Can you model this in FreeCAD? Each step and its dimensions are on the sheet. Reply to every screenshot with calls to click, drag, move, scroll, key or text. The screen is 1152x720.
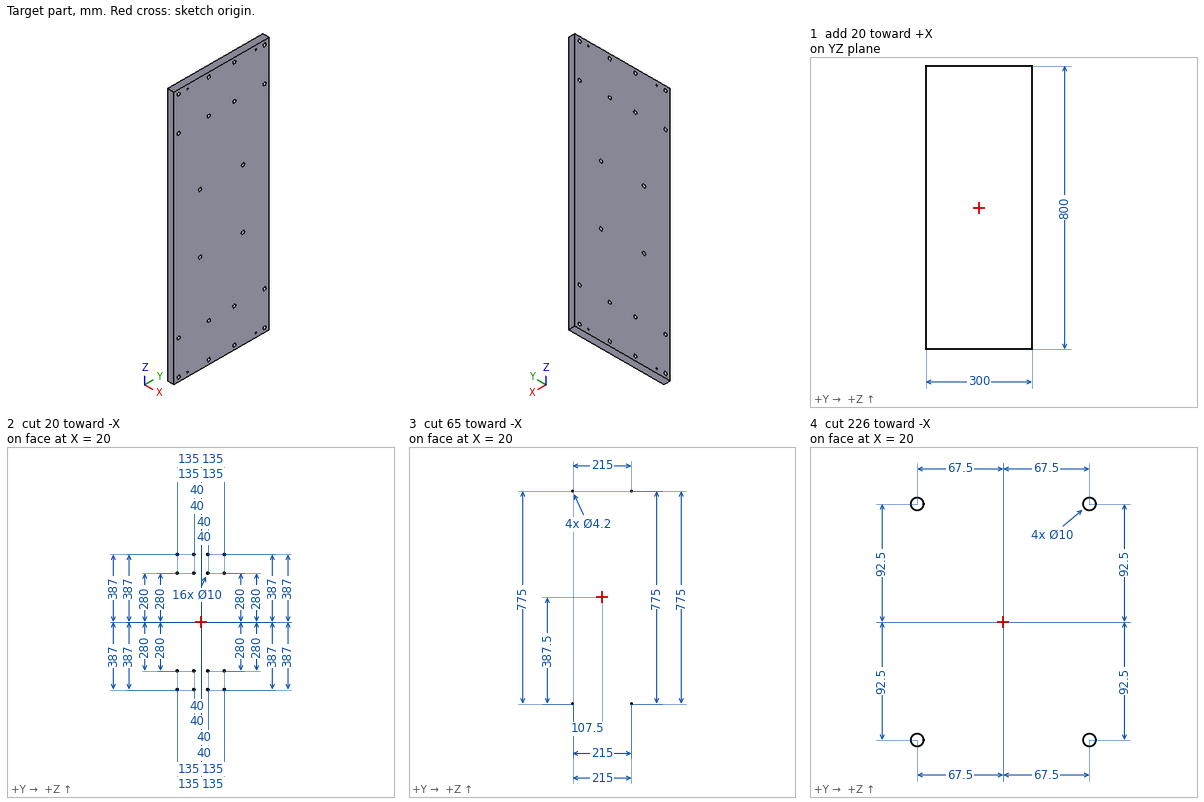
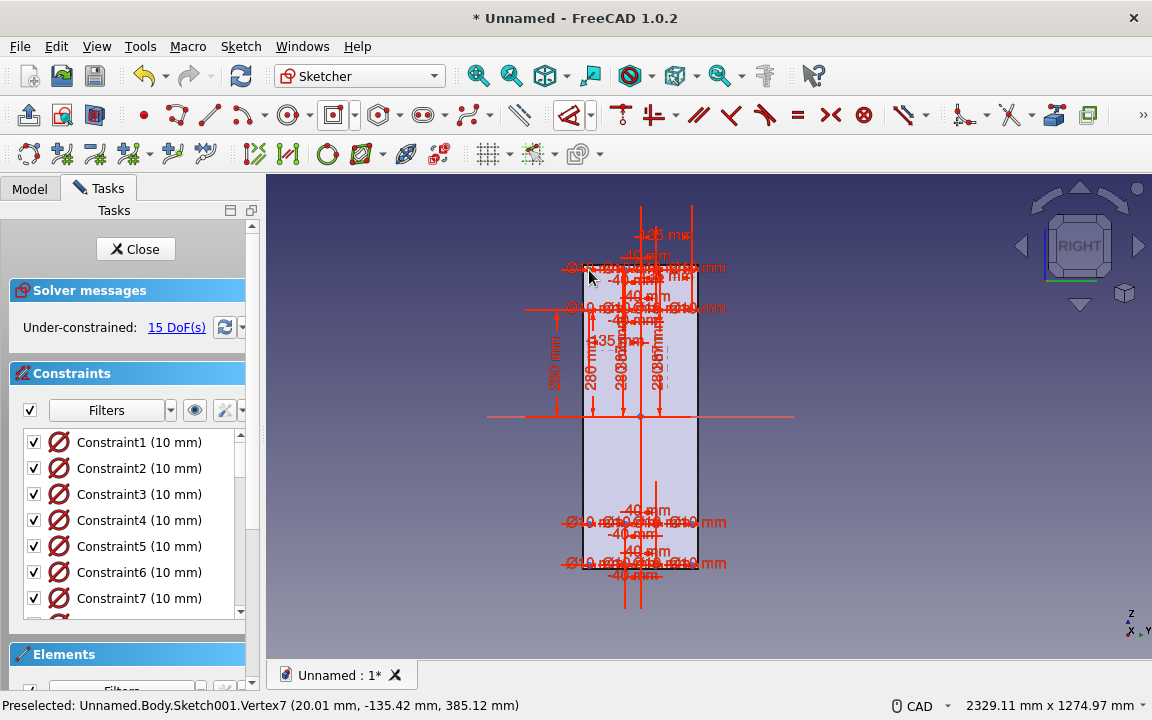
key(l)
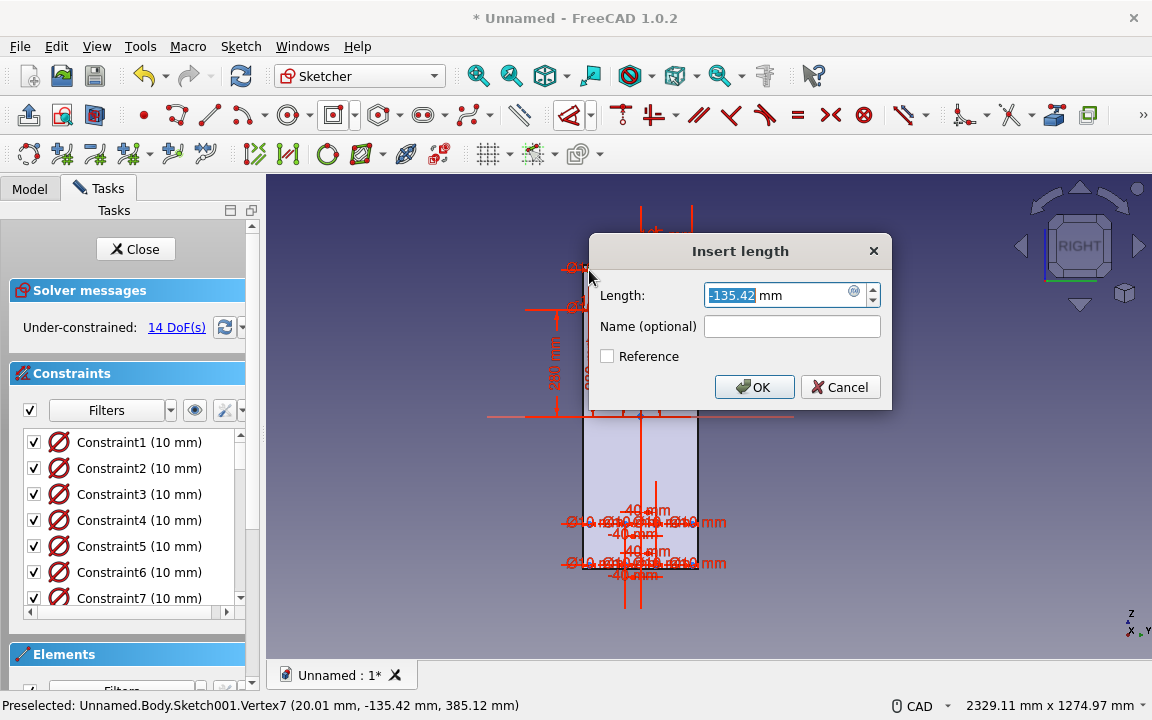
text(-135)
key(Return)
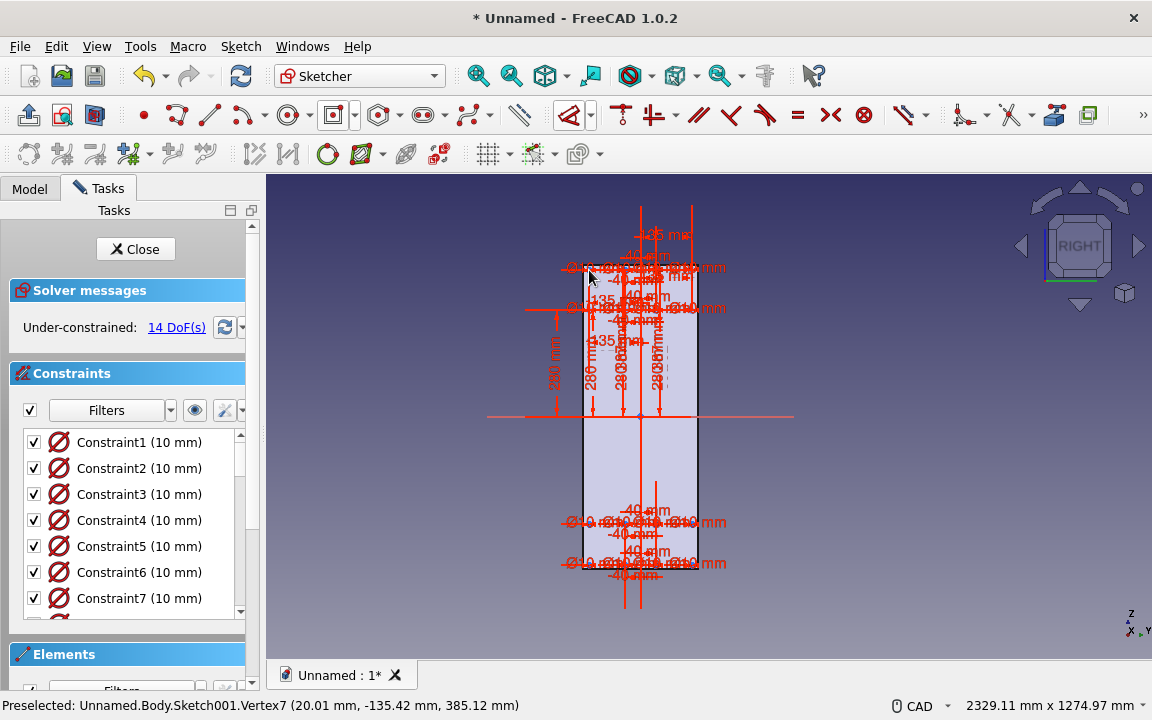
click(589, 270)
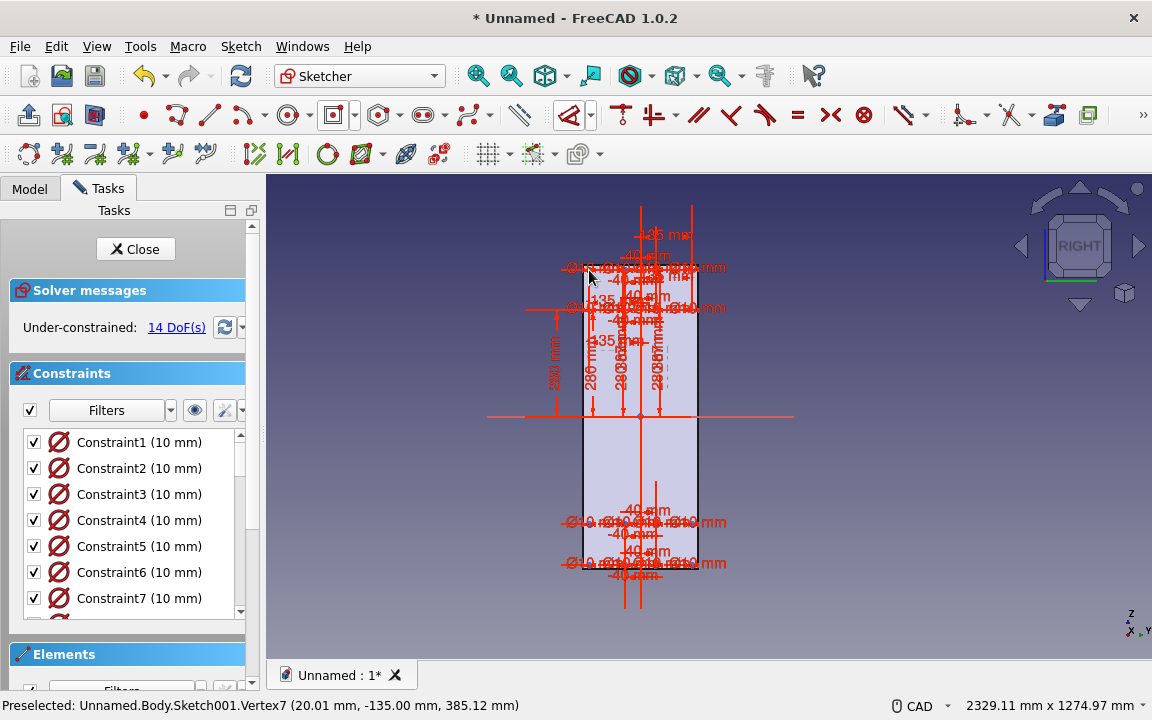
key(i)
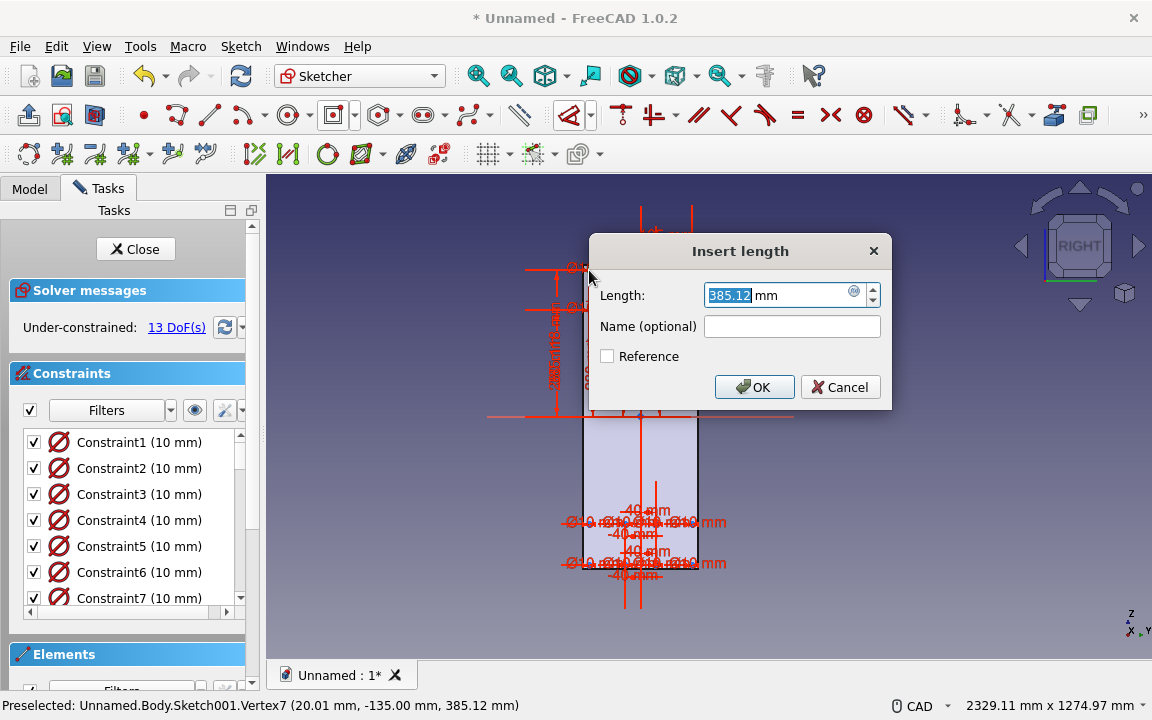
text(387)
key(Return)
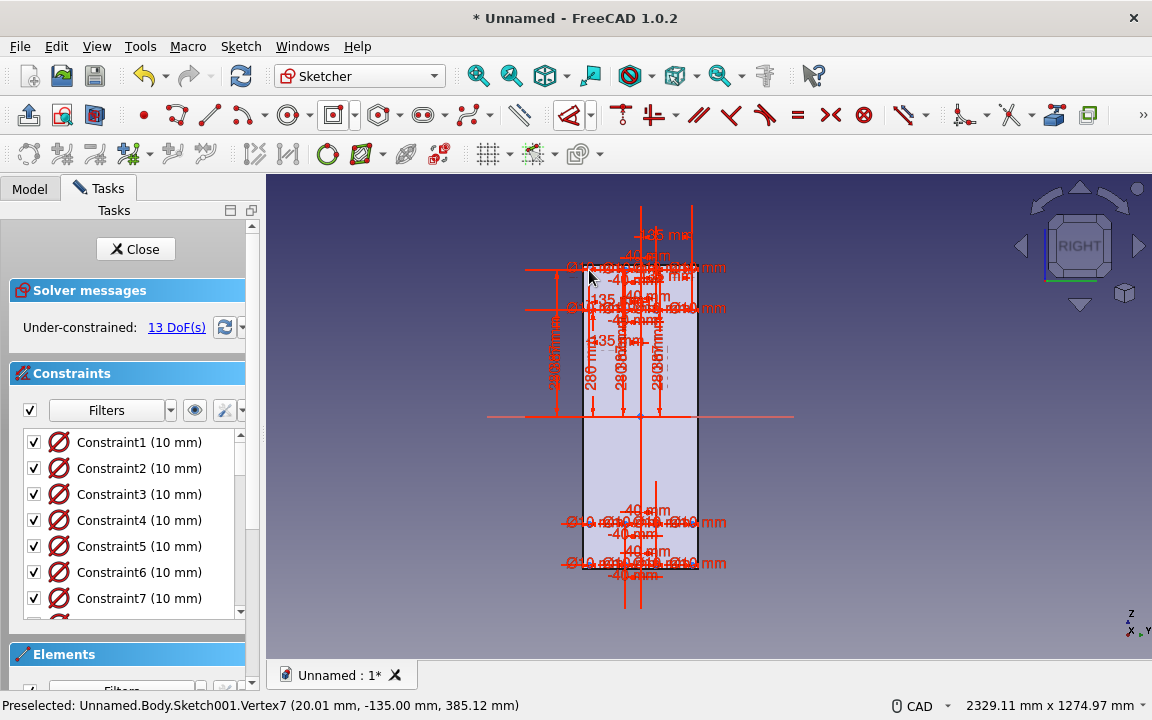
click(625, 270)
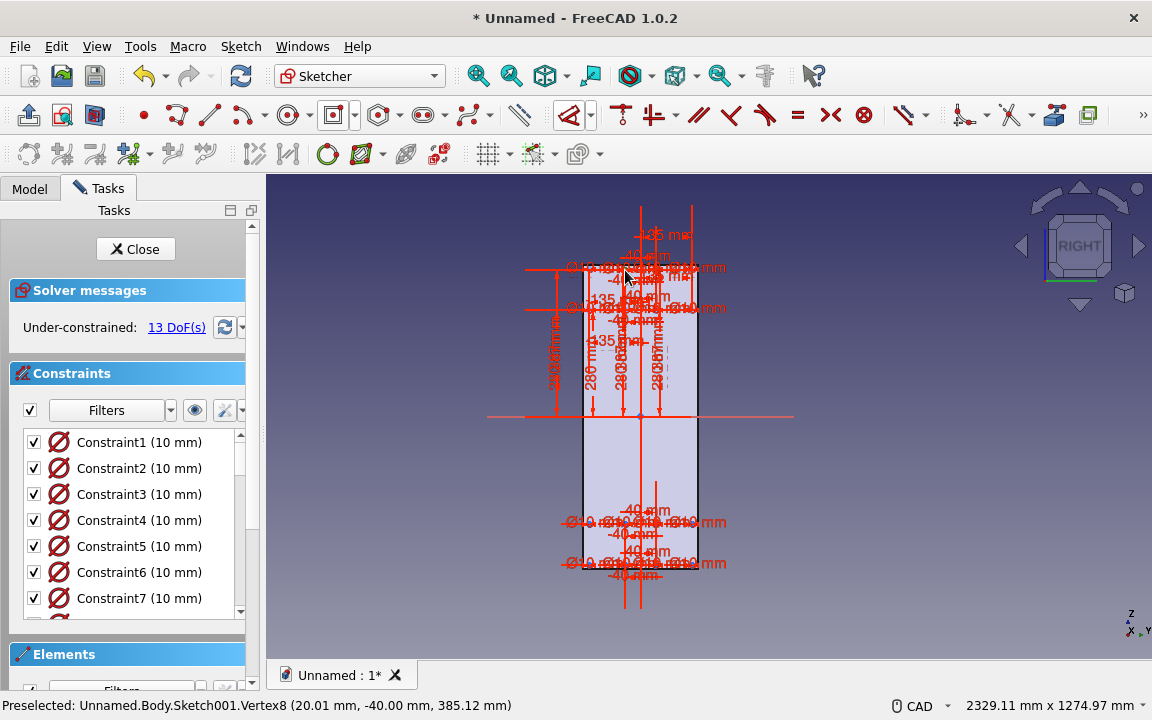
key(i)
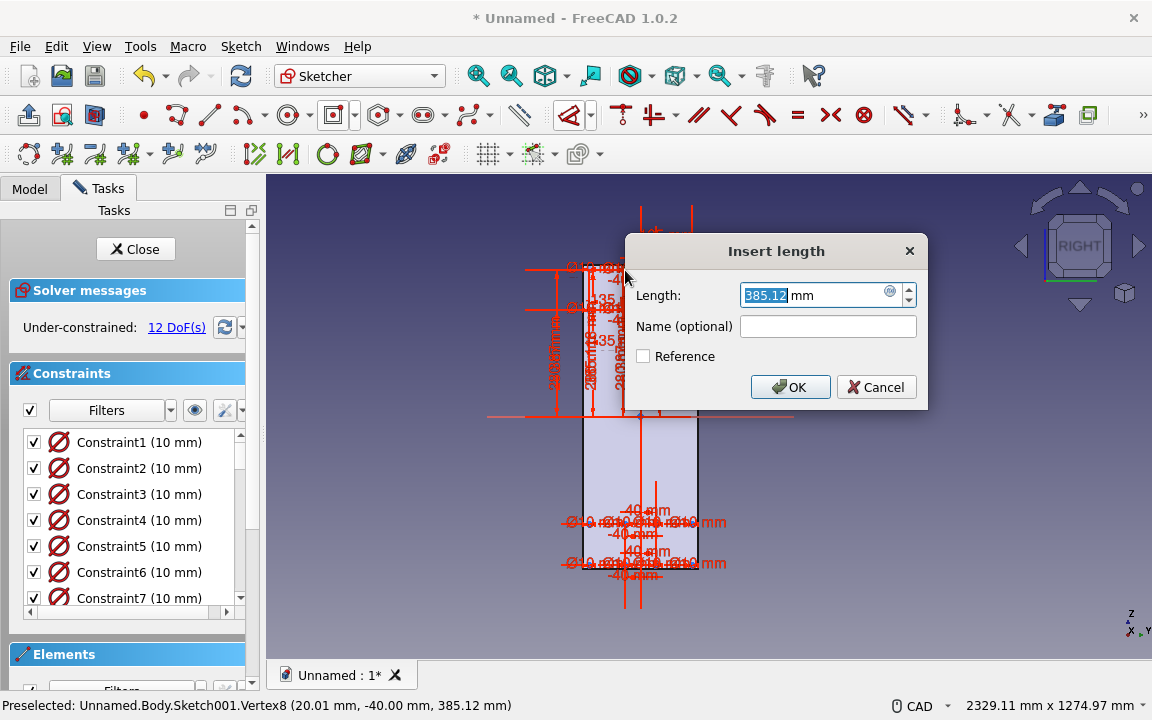
text(387)
key(Return)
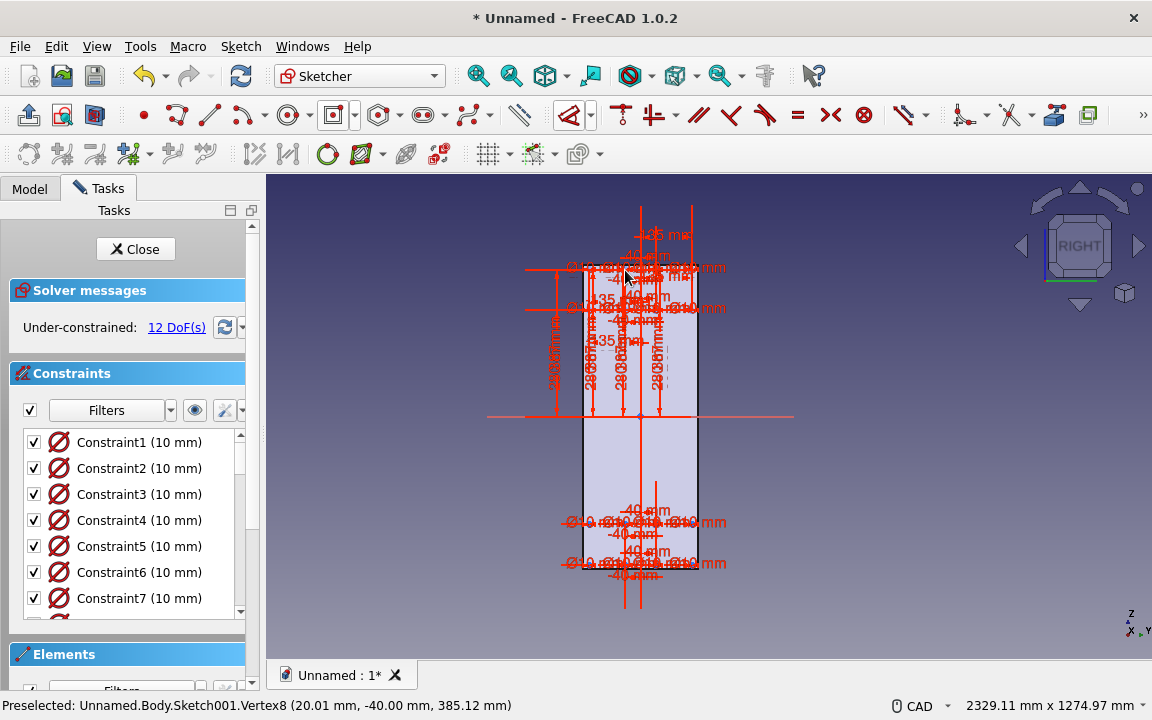
click(625, 524)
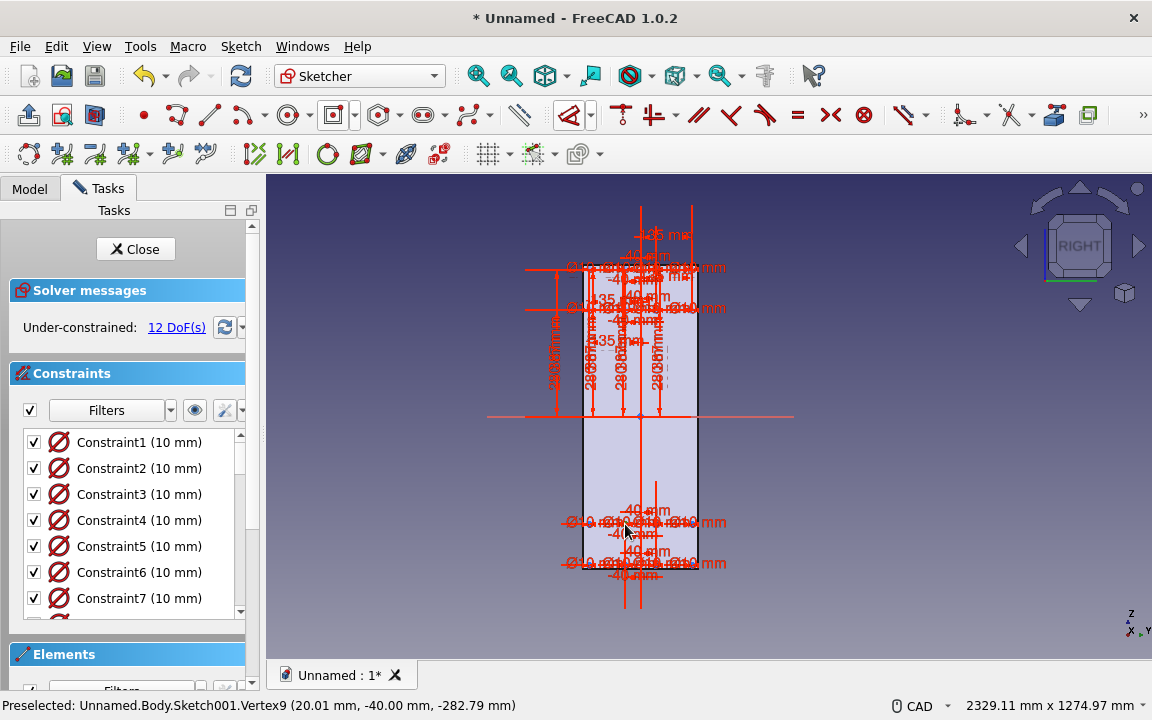
click(590, 116)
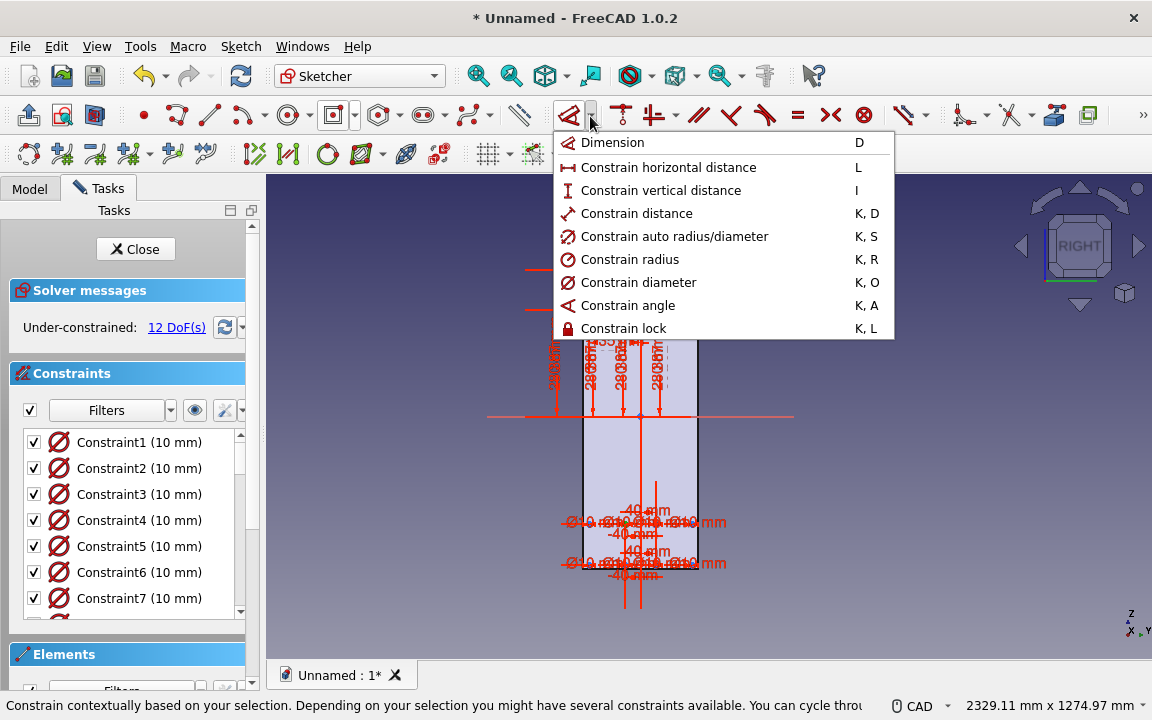
click(724, 190)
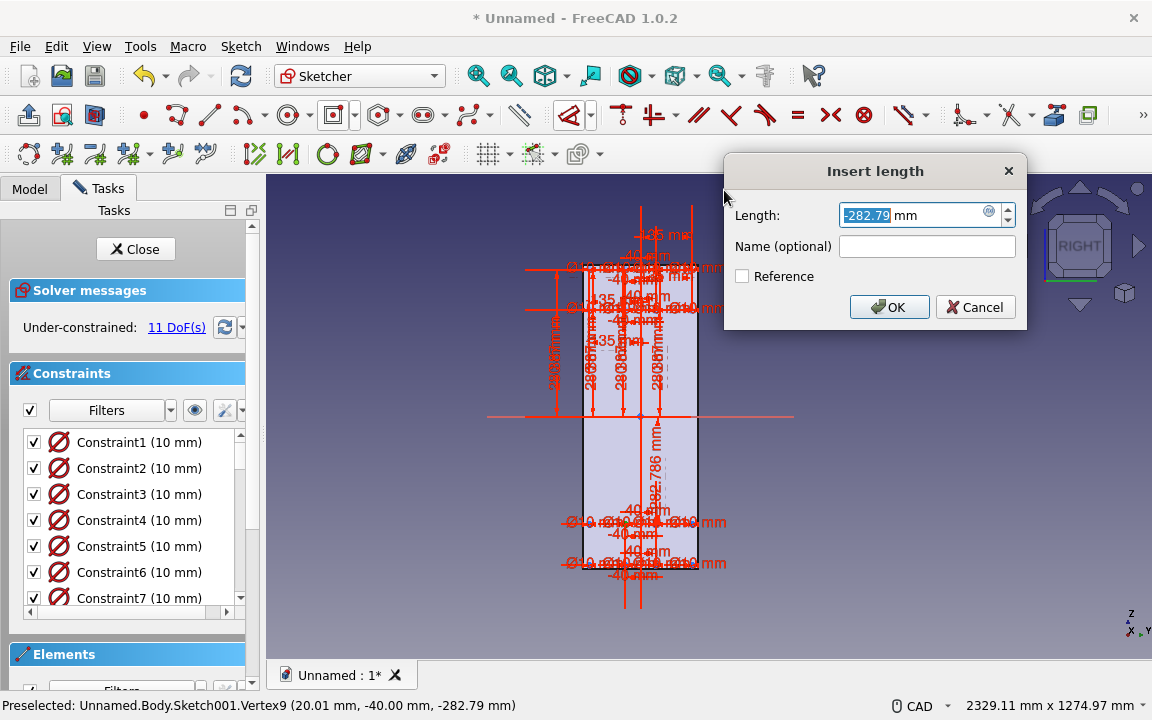
text(-280)
key(Return)